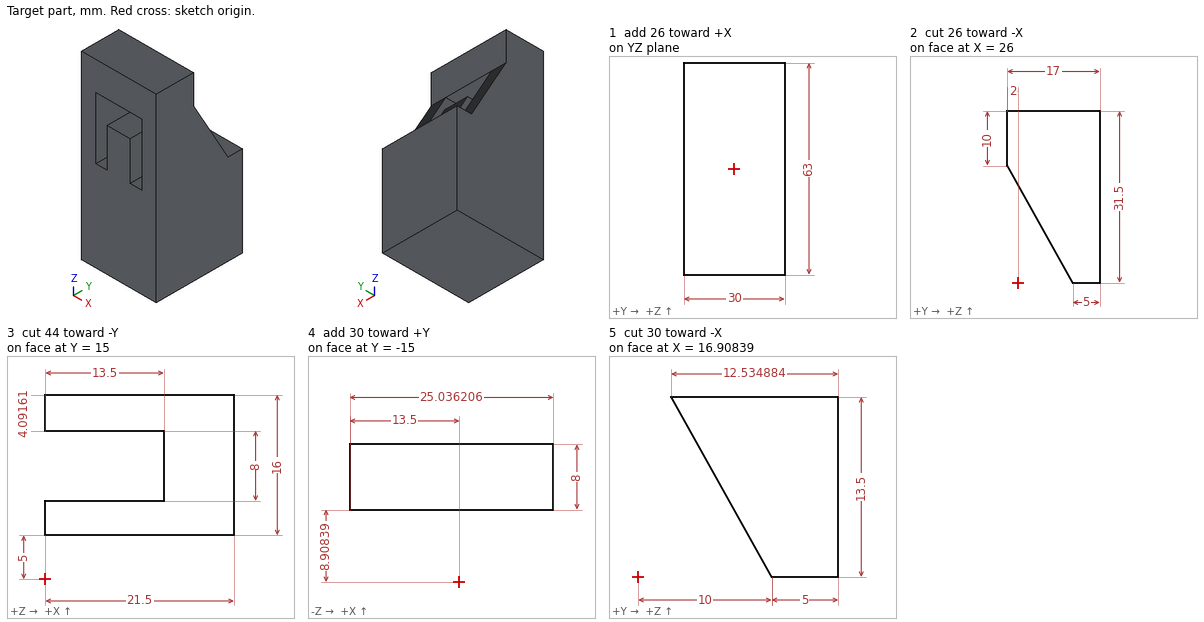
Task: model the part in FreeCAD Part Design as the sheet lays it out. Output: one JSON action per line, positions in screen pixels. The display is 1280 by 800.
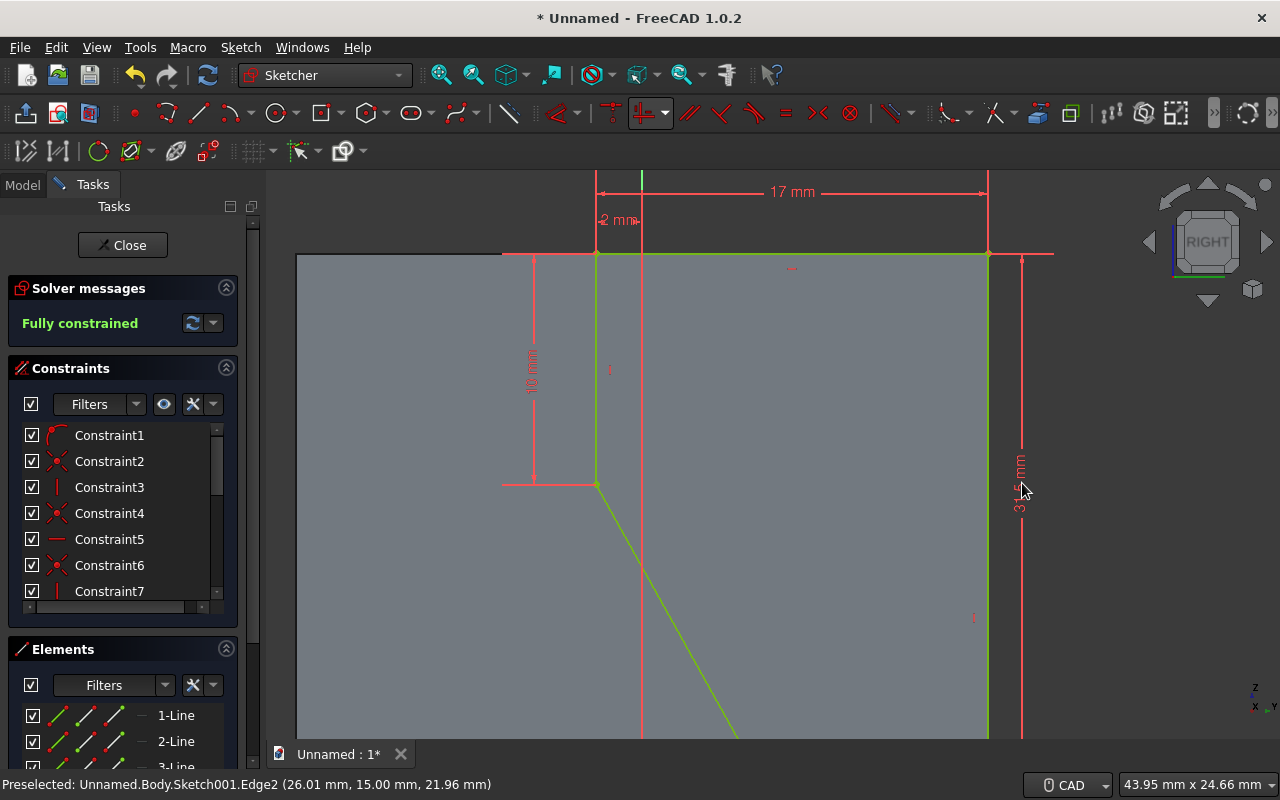
{"action": "left_click", "coordinate": [123, 245]}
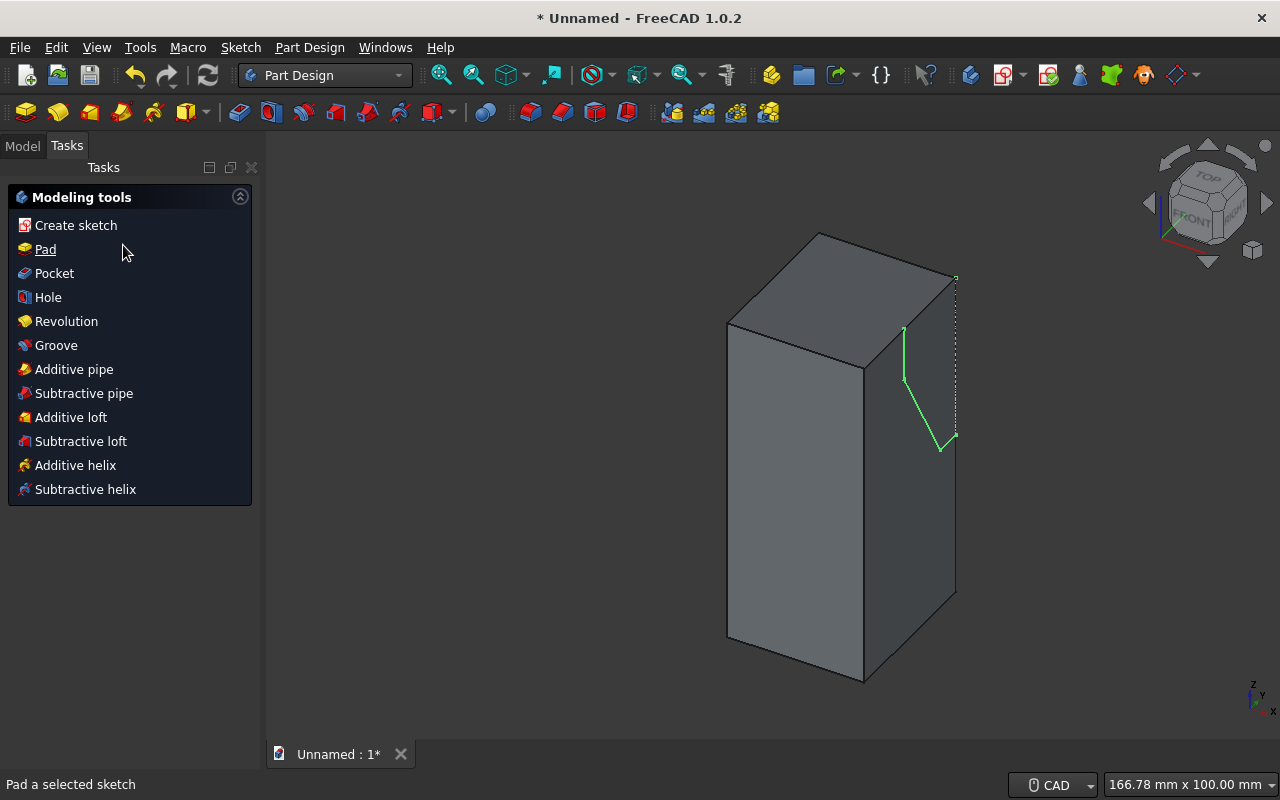
{"action": "left_click", "coordinate": [240, 112]}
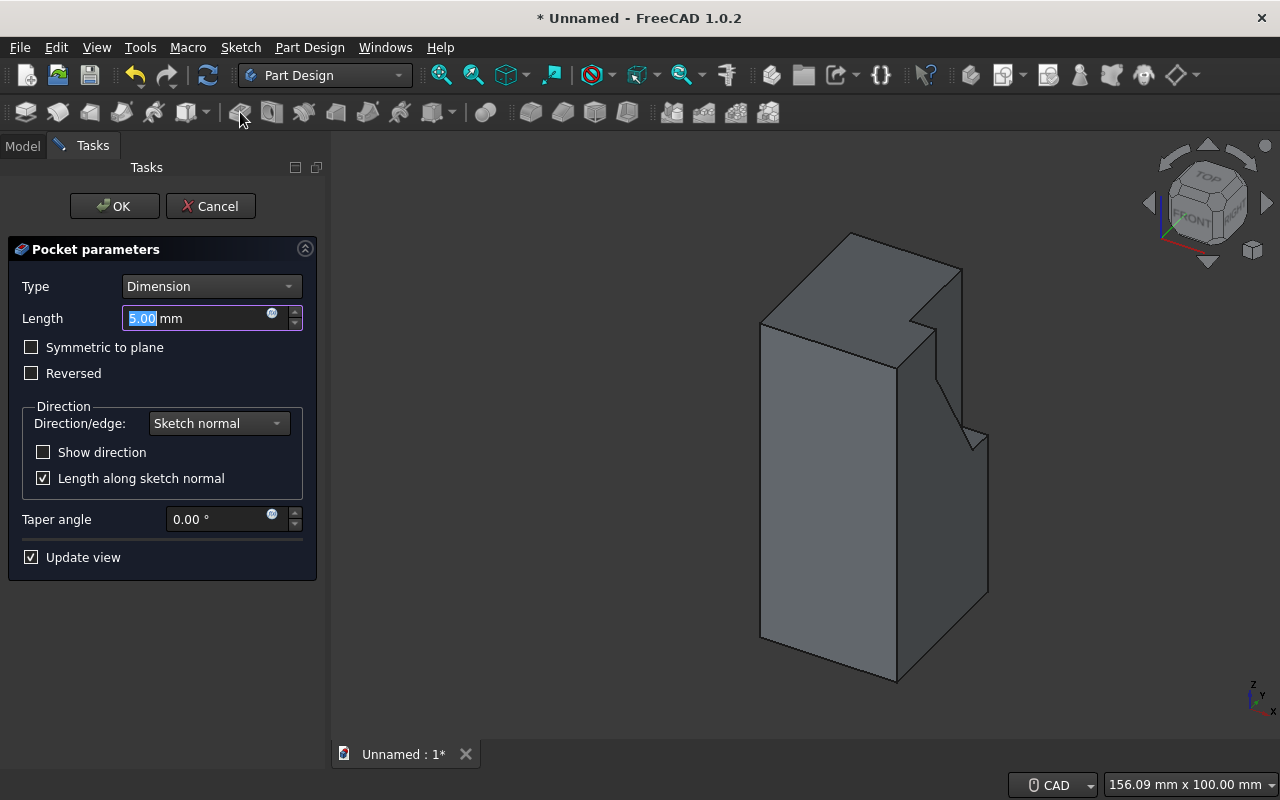
{"action": "type", "text": "26"}
{"action": "key", "text": "Tab"}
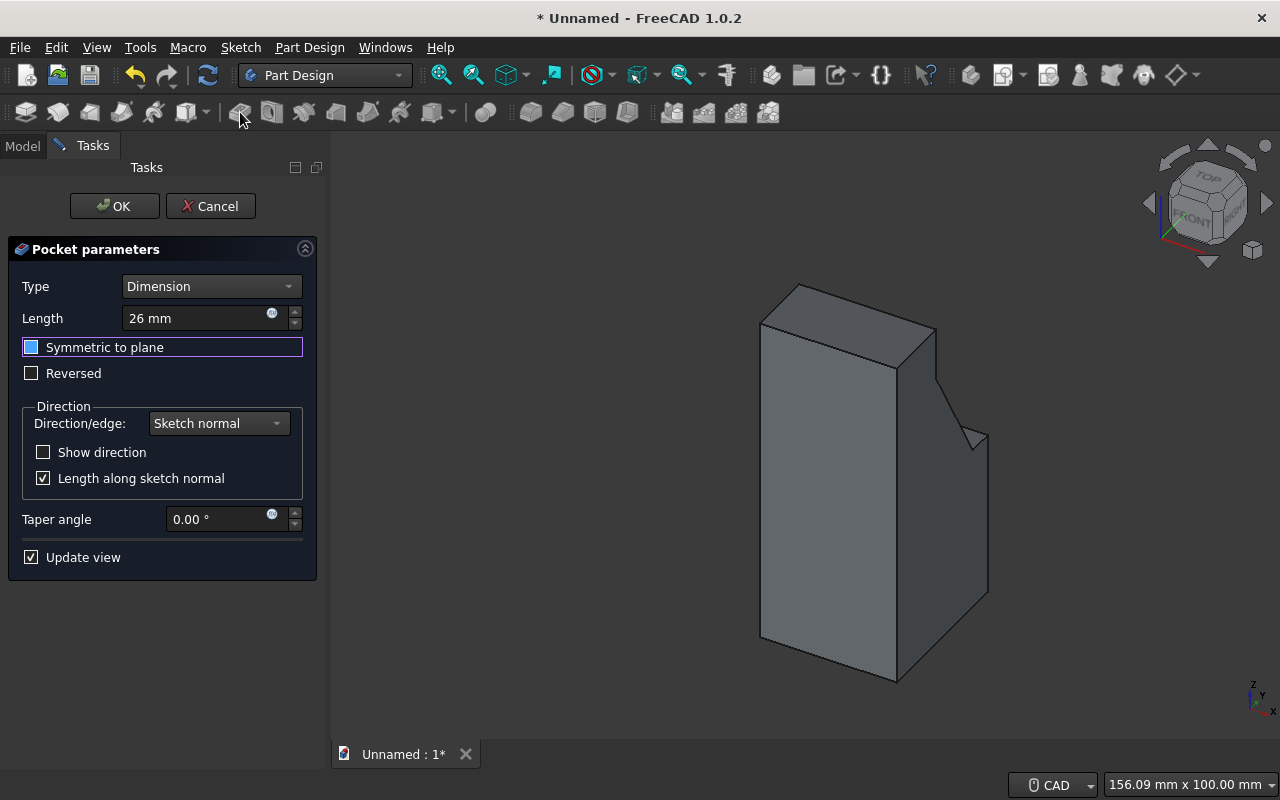
{"action": "left_click", "coordinate": [115, 206]}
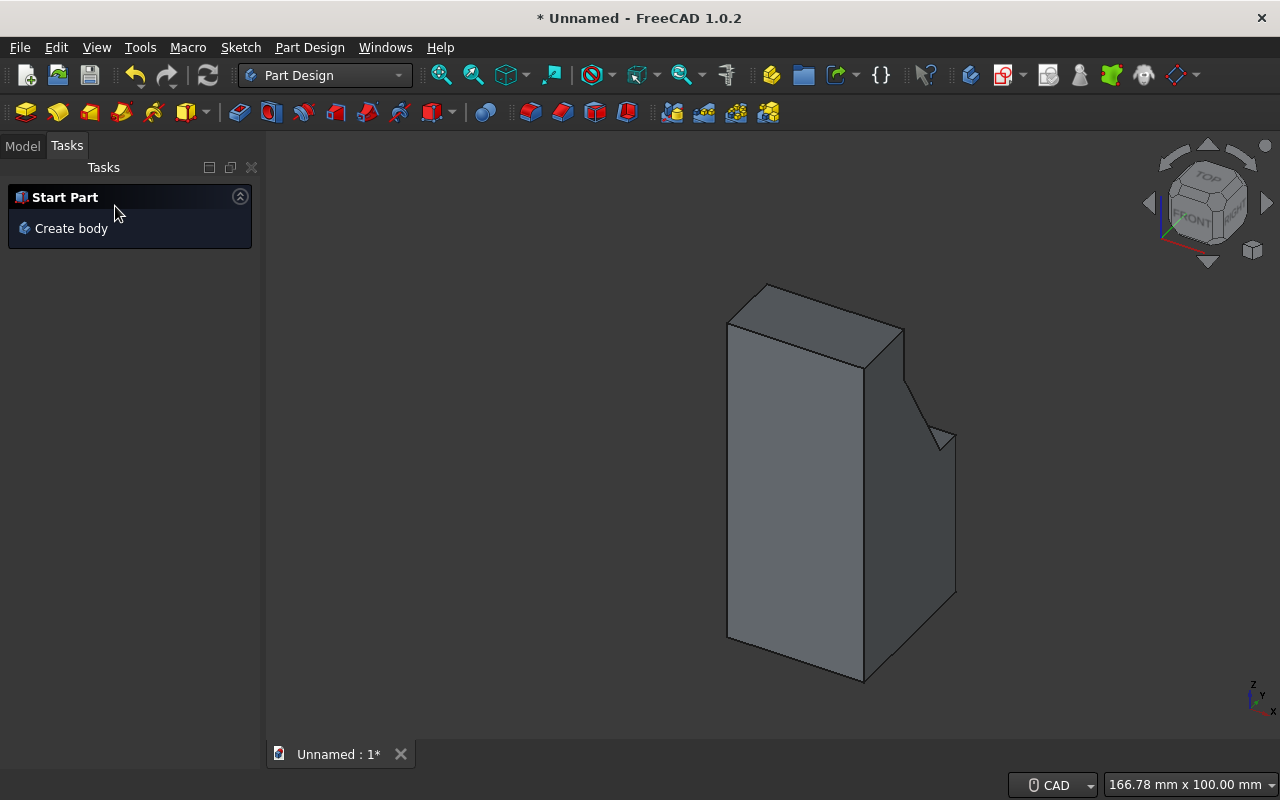
{"action": "key", "text": "4"}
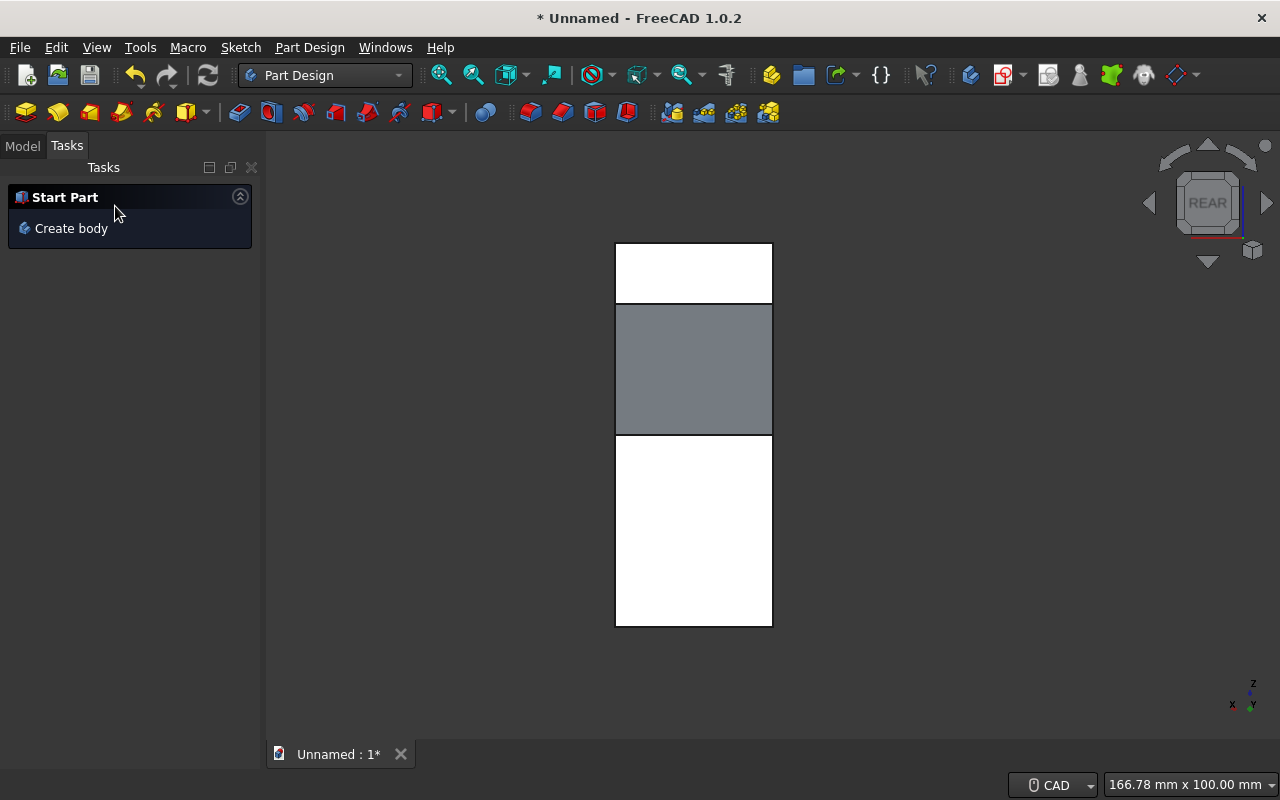
{"action": "left_click", "coordinate": [694, 530]}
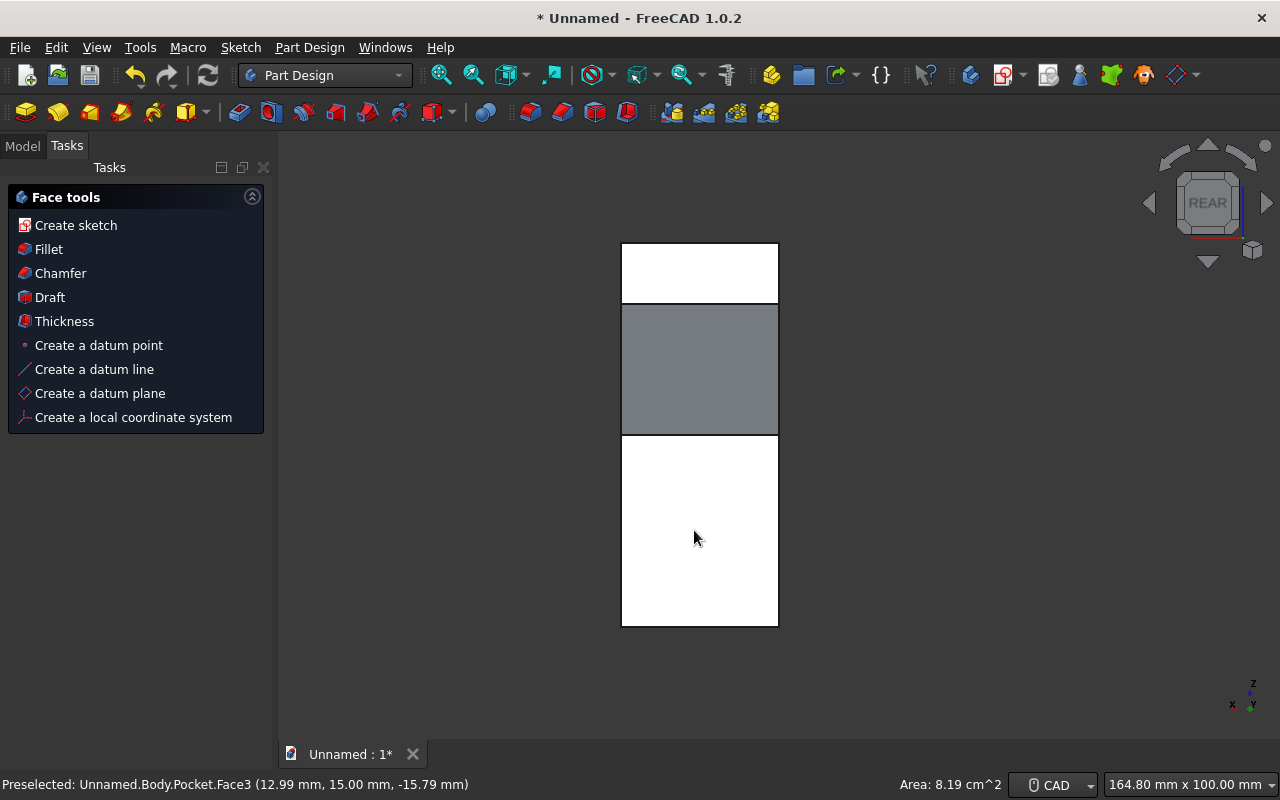
{"action": "left_click", "coordinate": [1004, 76]}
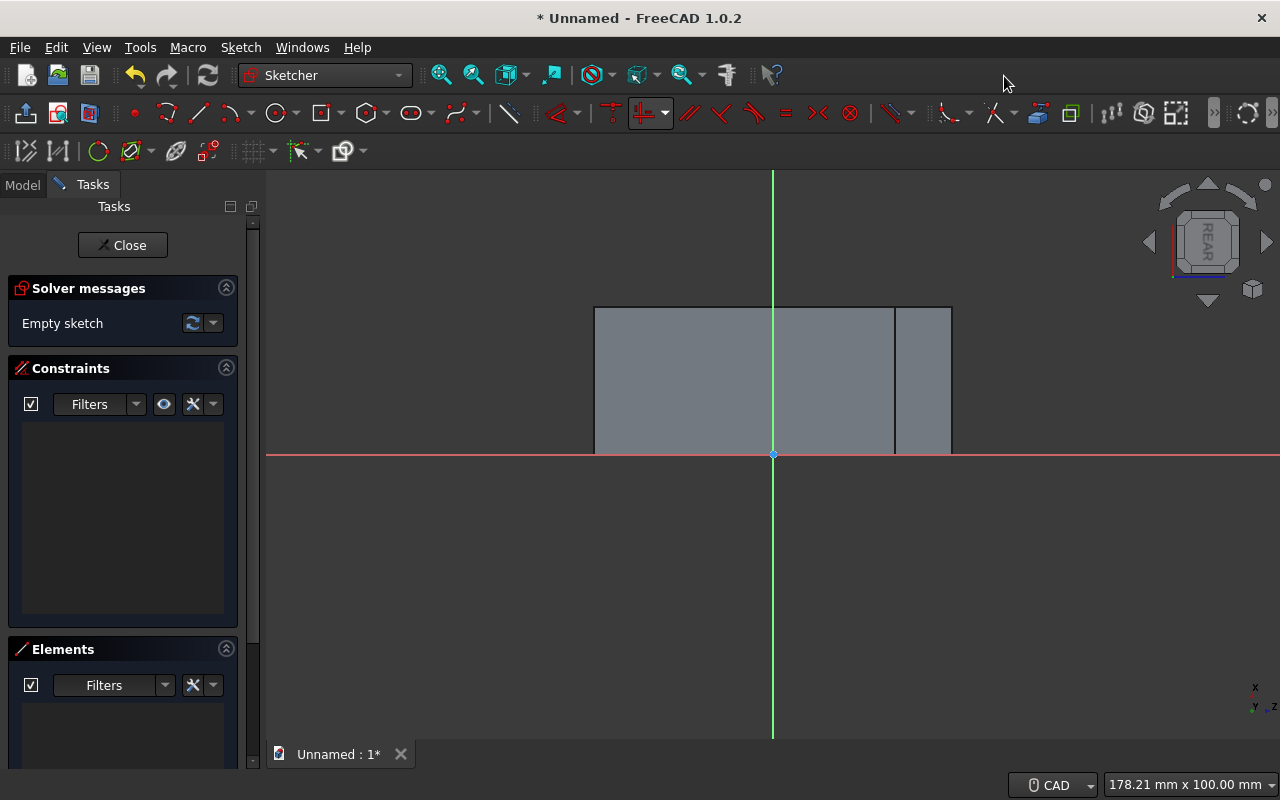
{"action": "scroll", "coordinate": [890, 369], "scroll_direction": "up", "scroll_amount": 6}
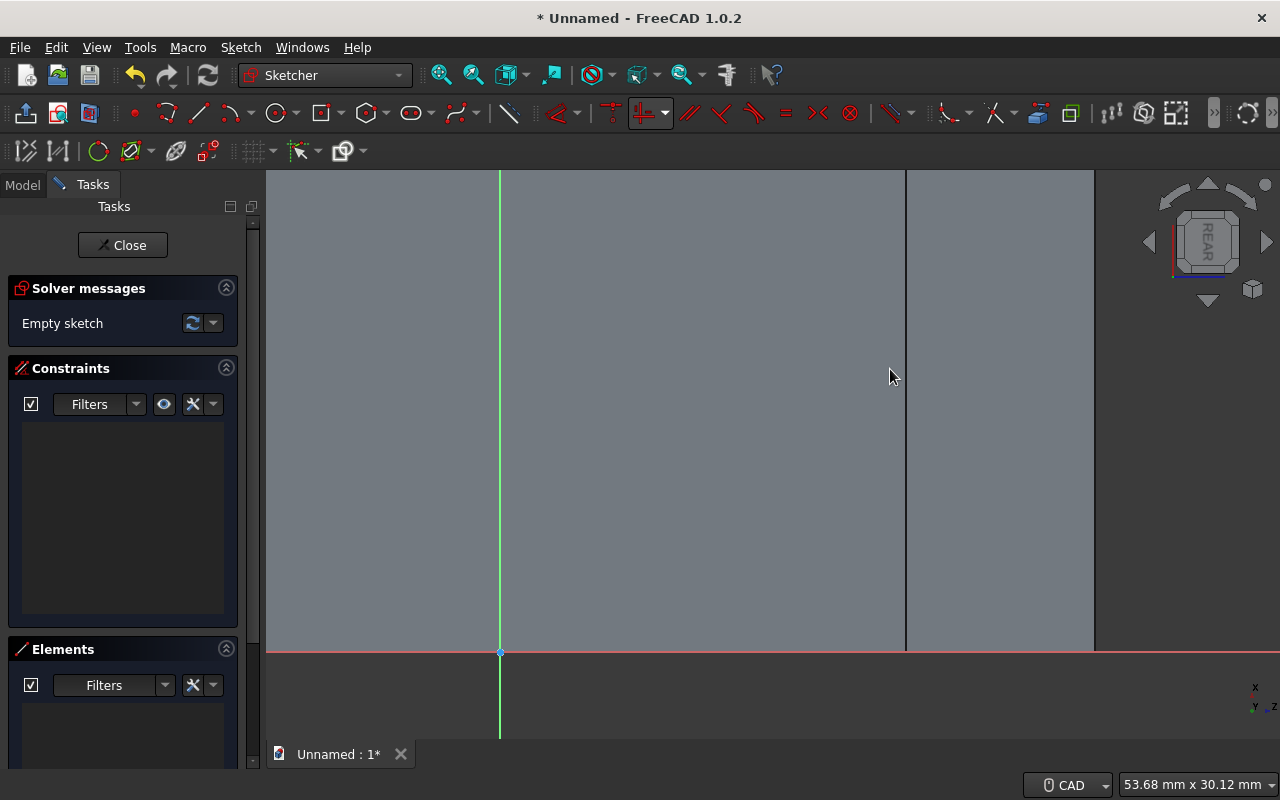
{"action": "left_click", "coordinate": [168, 114]}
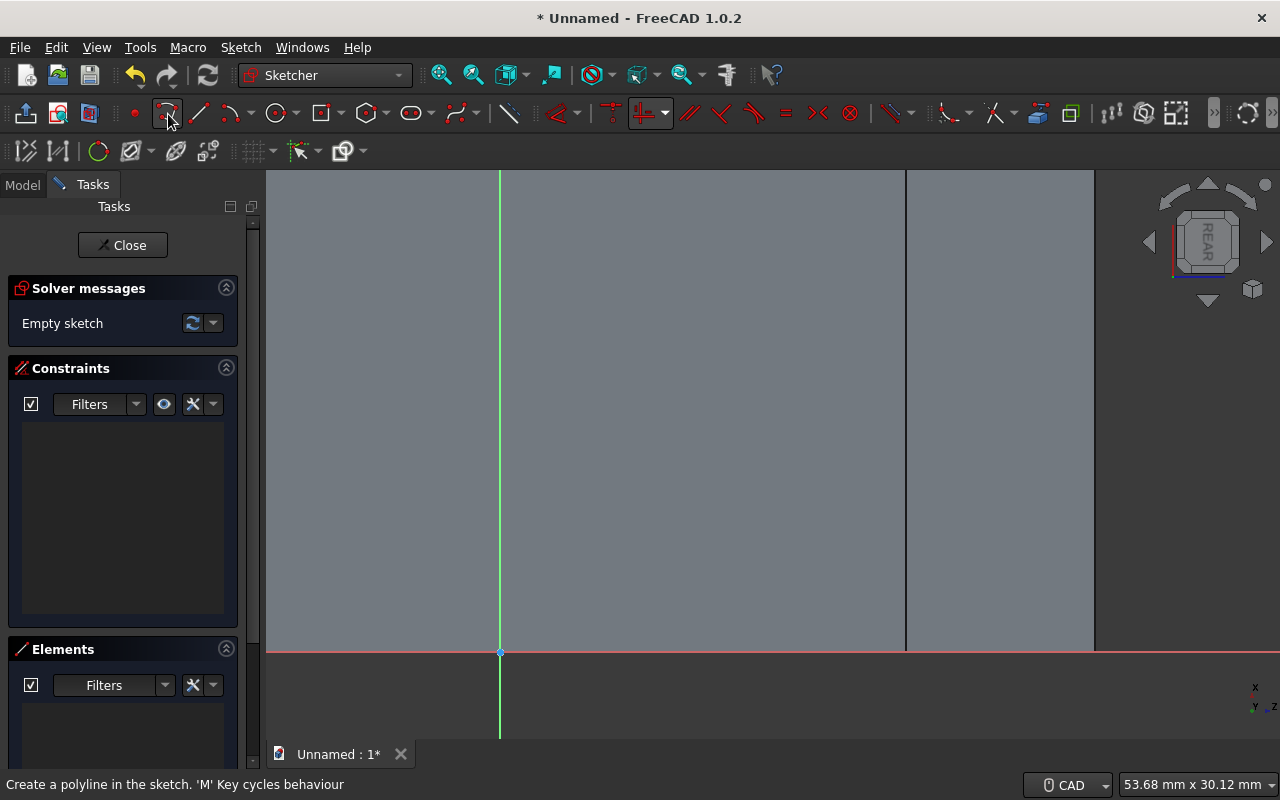
{"action": "left_click", "coordinate": [500, 558]}
{"action": "left_click", "coordinate": [906, 558]}
{"action": "left_click", "coordinate": [906, 255]}
{"action": "left_click", "coordinate": [500, 255]}
{"action": "left_click", "coordinate": [509, 333]}
{"action": "left_click", "coordinate": [755, 333]}
{"action": "left_click", "coordinate": [755, 484]}
{"action": "left_click", "coordinate": [509, 484]}
{"action": "left_click", "coordinate": [500, 559]}
{"action": "key", "text": "Escape"}
{"action": "key", "text": "Escape"}